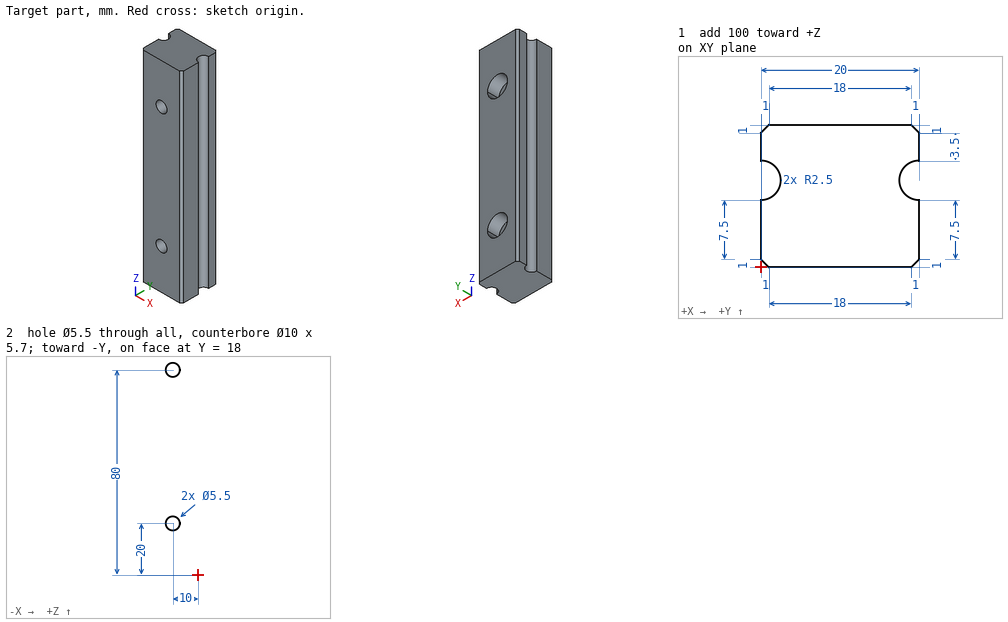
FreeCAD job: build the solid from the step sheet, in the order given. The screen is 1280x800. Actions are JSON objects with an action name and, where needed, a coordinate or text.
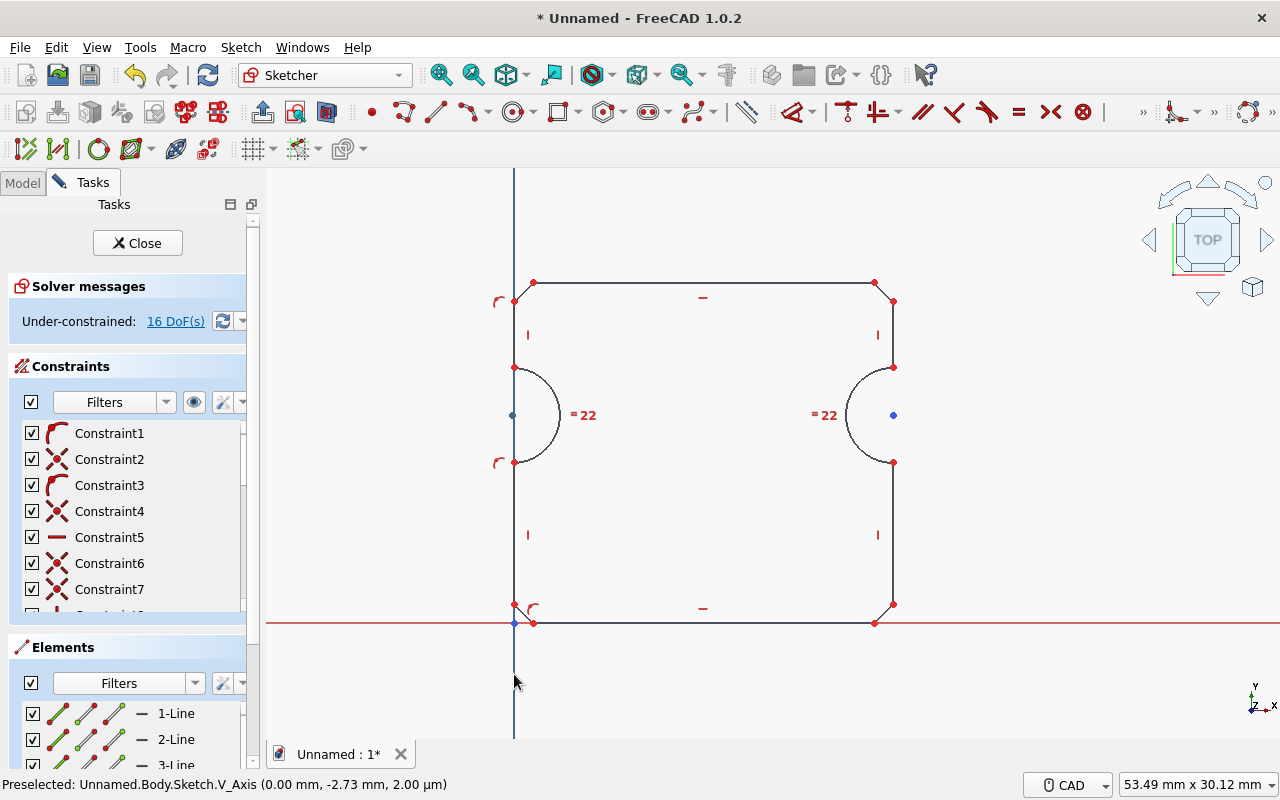
{"action": "left_click", "coordinate": [846, 112]}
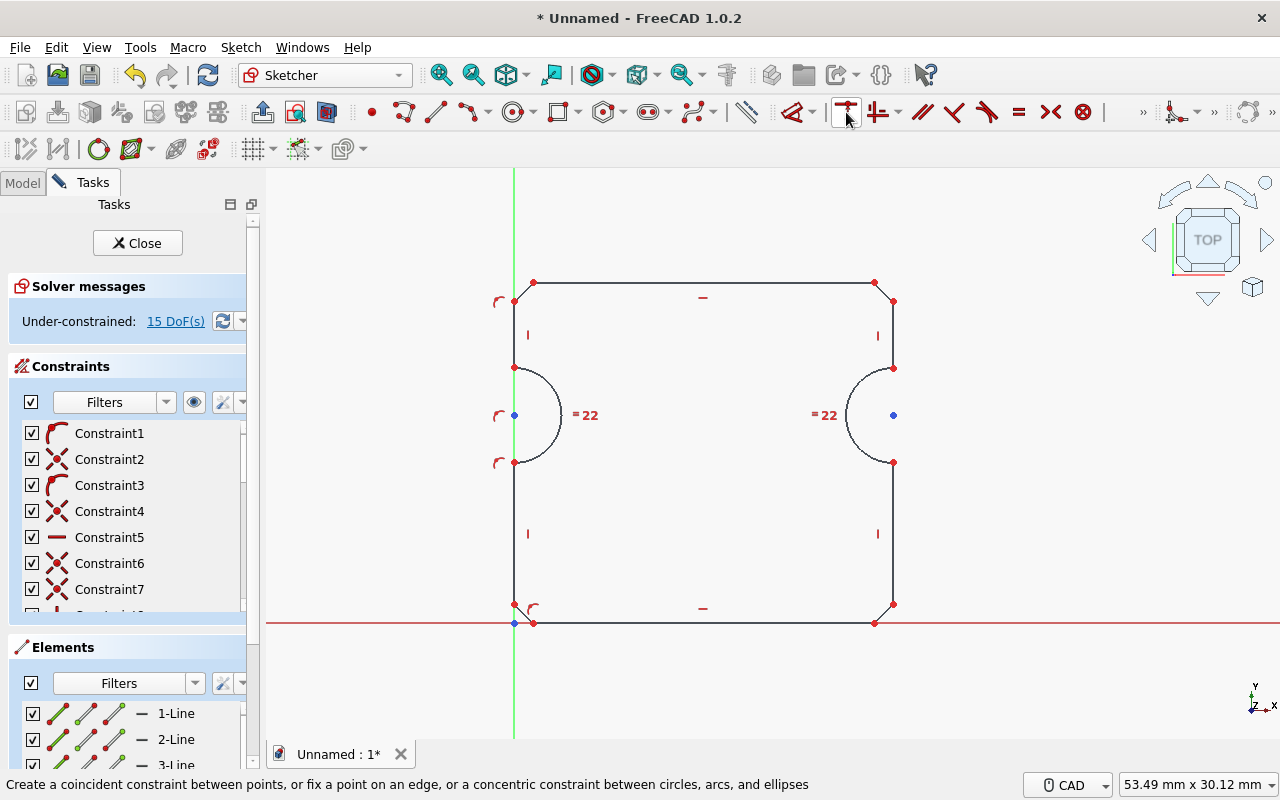
{"action": "left_click", "coordinate": [855, 388]}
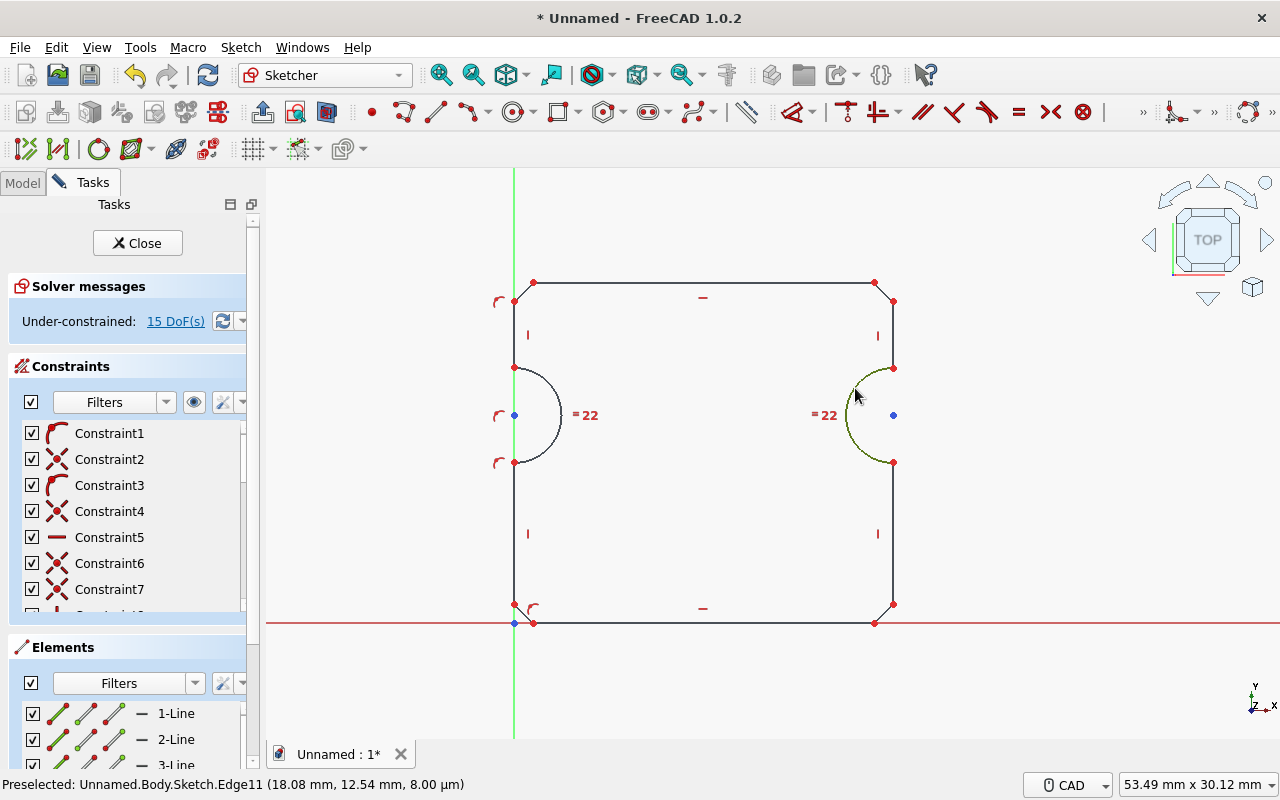
{"action": "key", "text": "k r"}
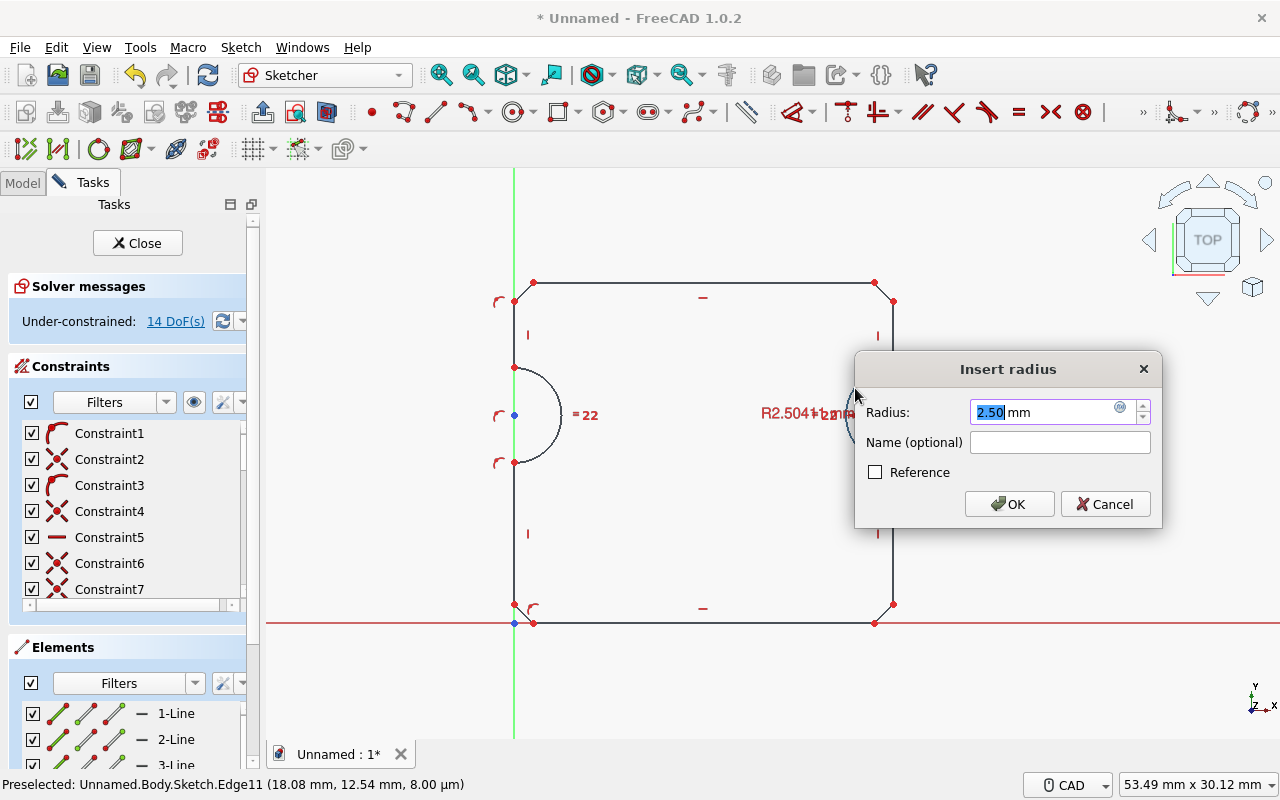
{"action": "type", "text": "2.5"}
{"action": "key", "text": "Return"}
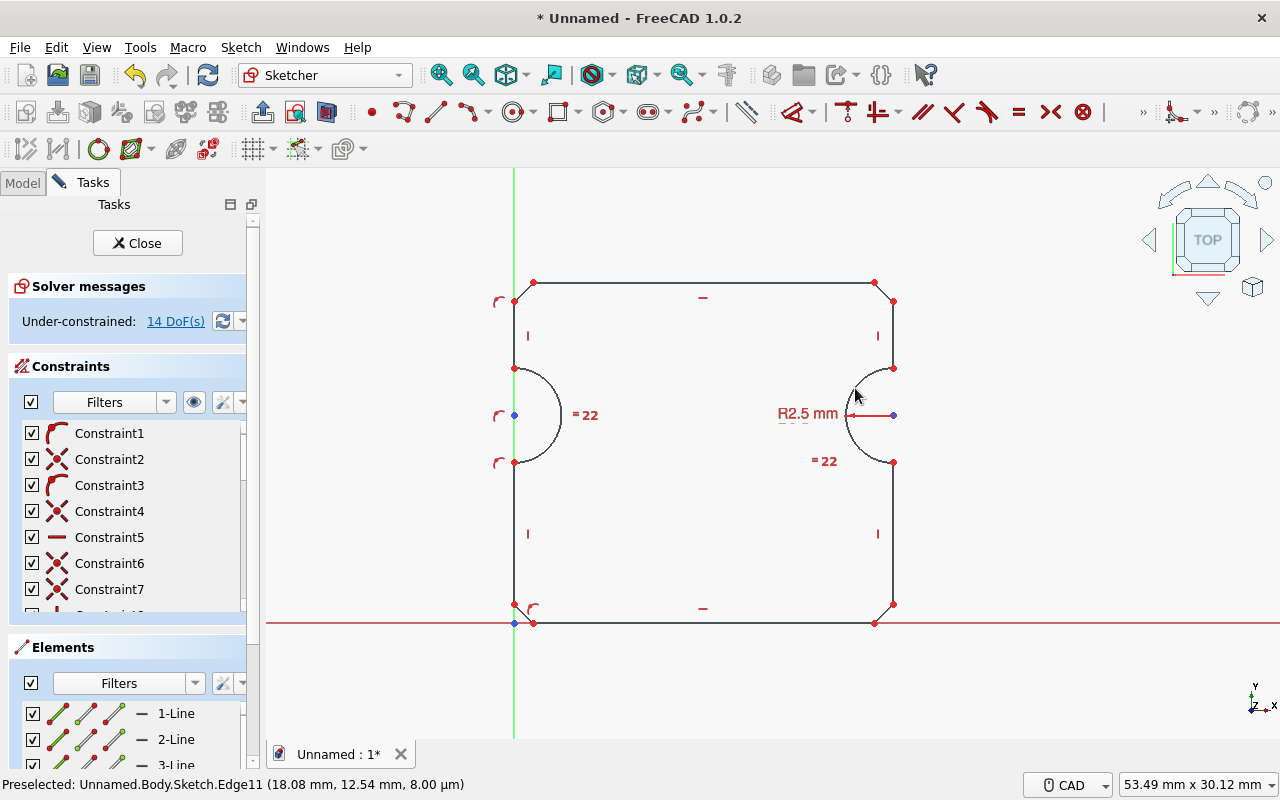
{"action": "left_click", "coordinate": [635, 623]}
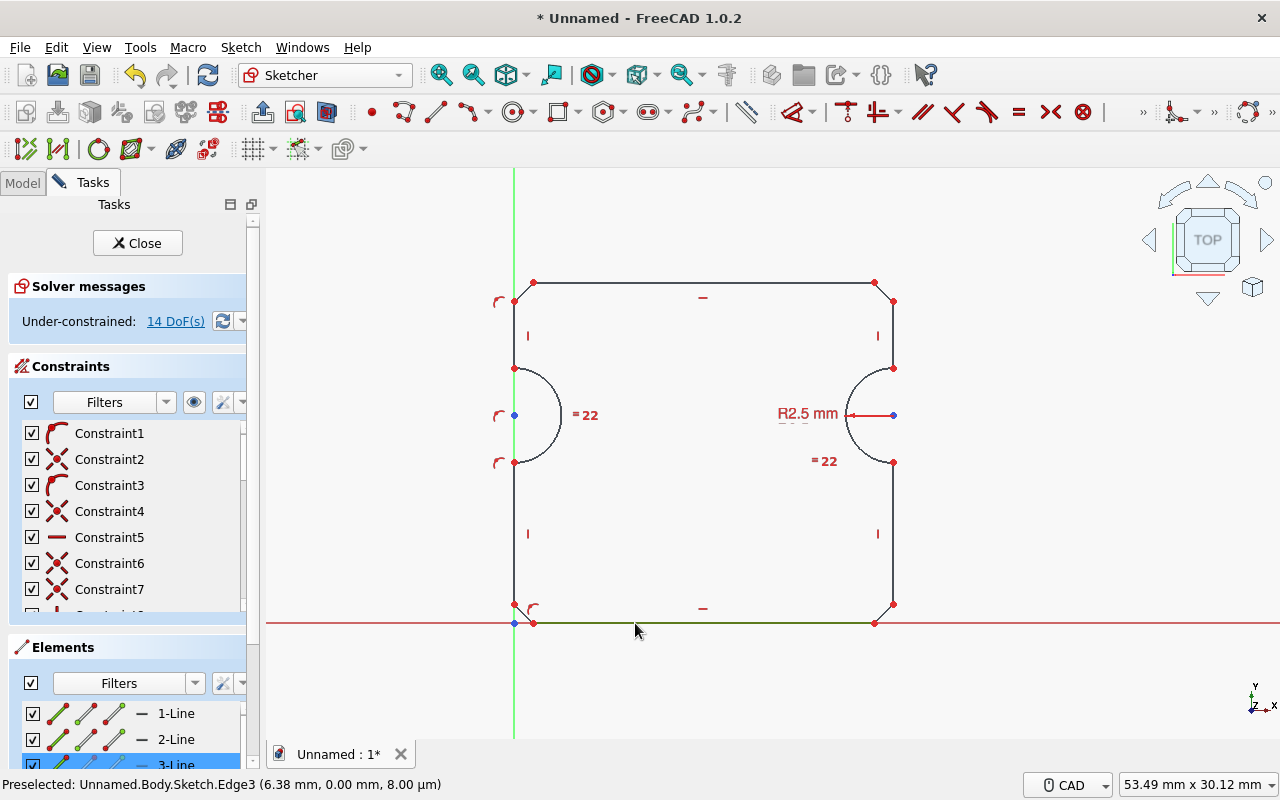
{"action": "left_click", "coordinate": [814, 112]}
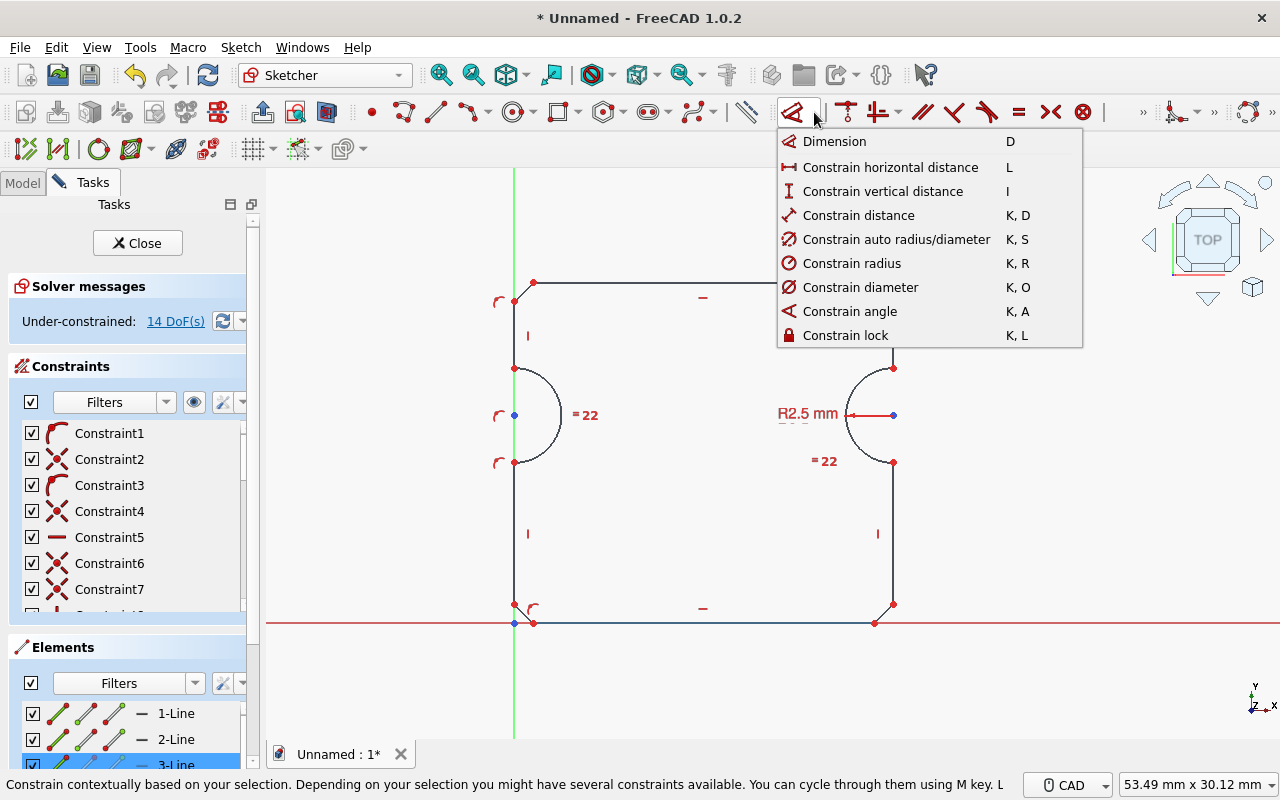
{"action": "left_click", "coordinate": [930, 167]}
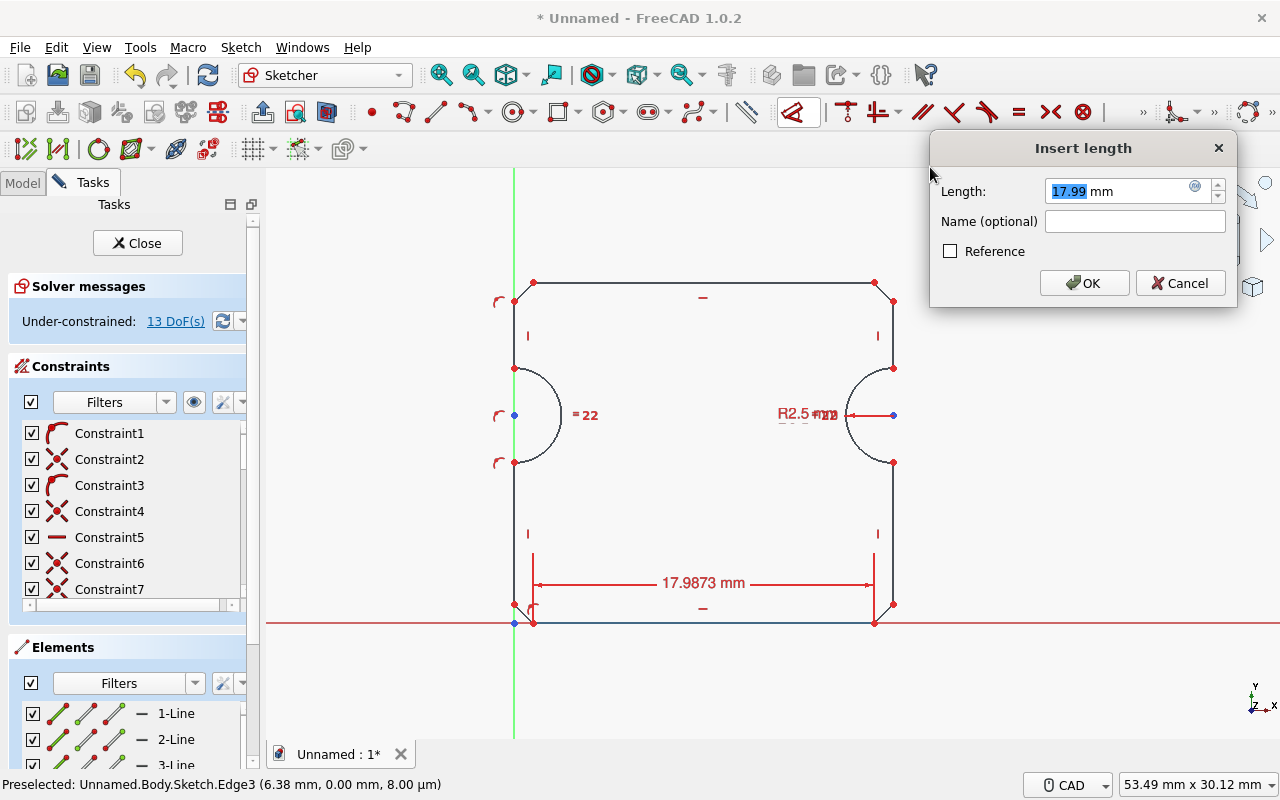
{"action": "type", "text": "18"}
{"action": "key", "text": "Return"}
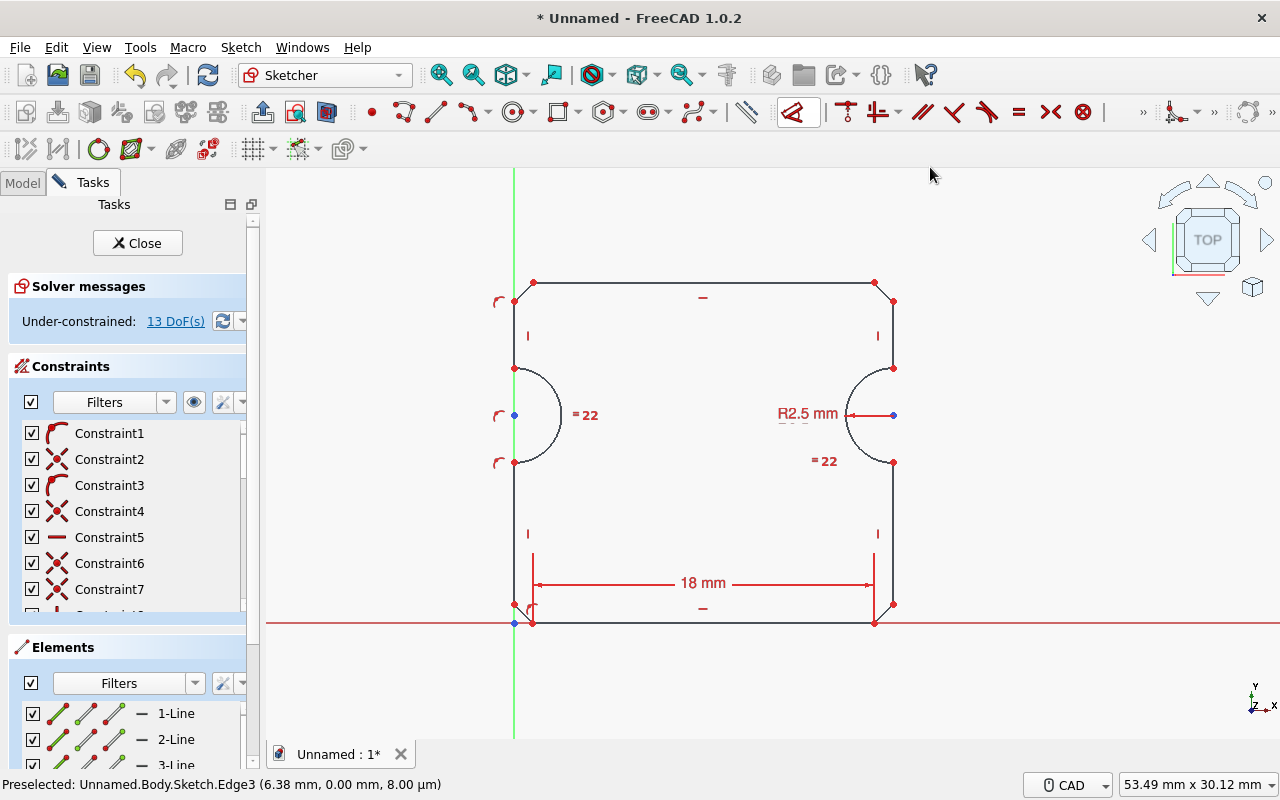
{"action": "left_click", "coordinate": [772, 283]}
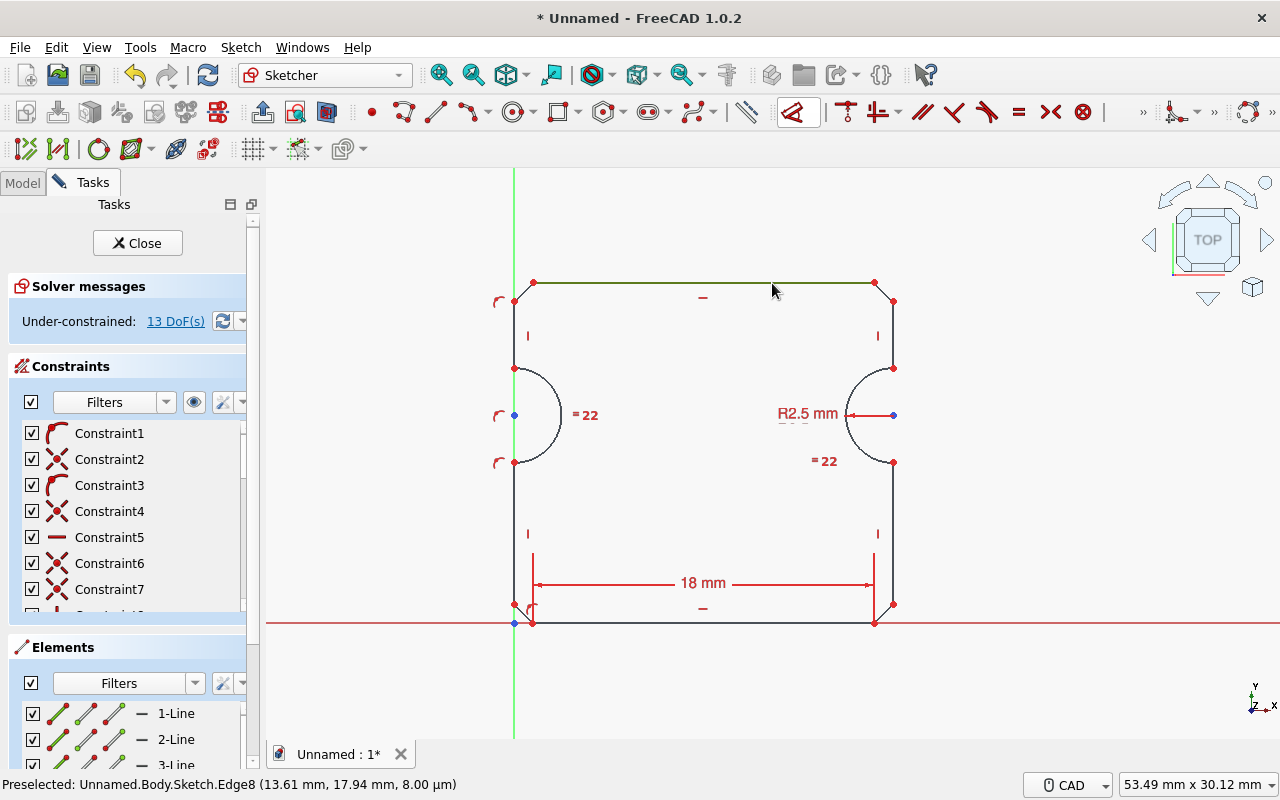
{"action": "left_click", "coordinate": [814, 112]}